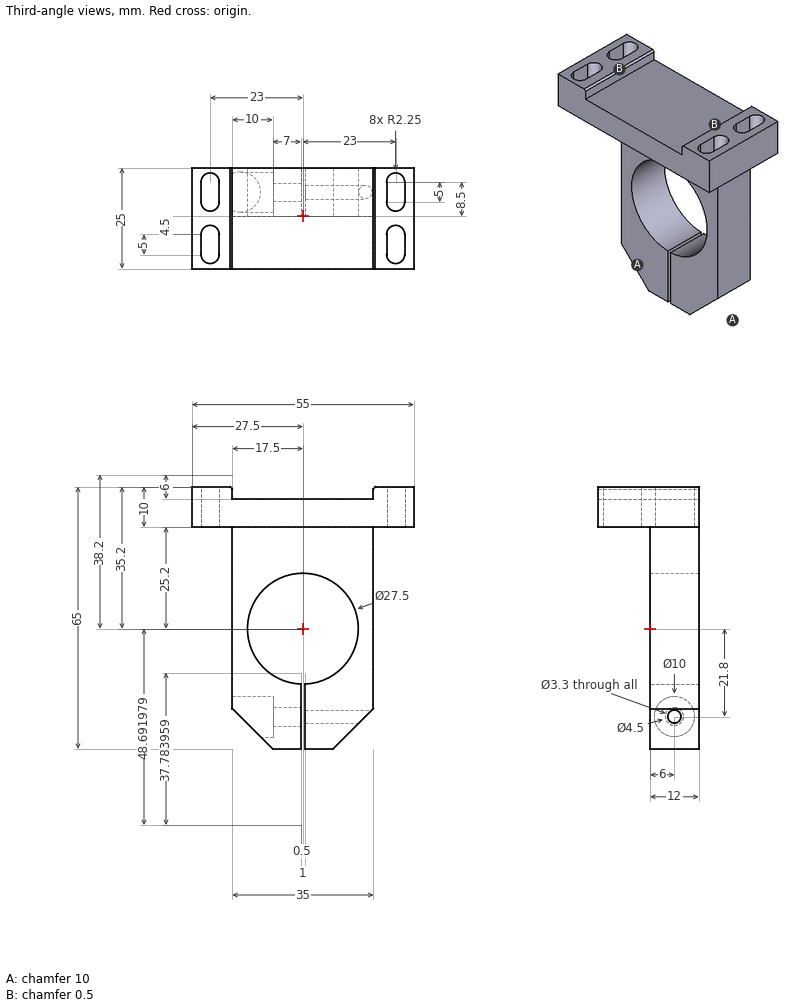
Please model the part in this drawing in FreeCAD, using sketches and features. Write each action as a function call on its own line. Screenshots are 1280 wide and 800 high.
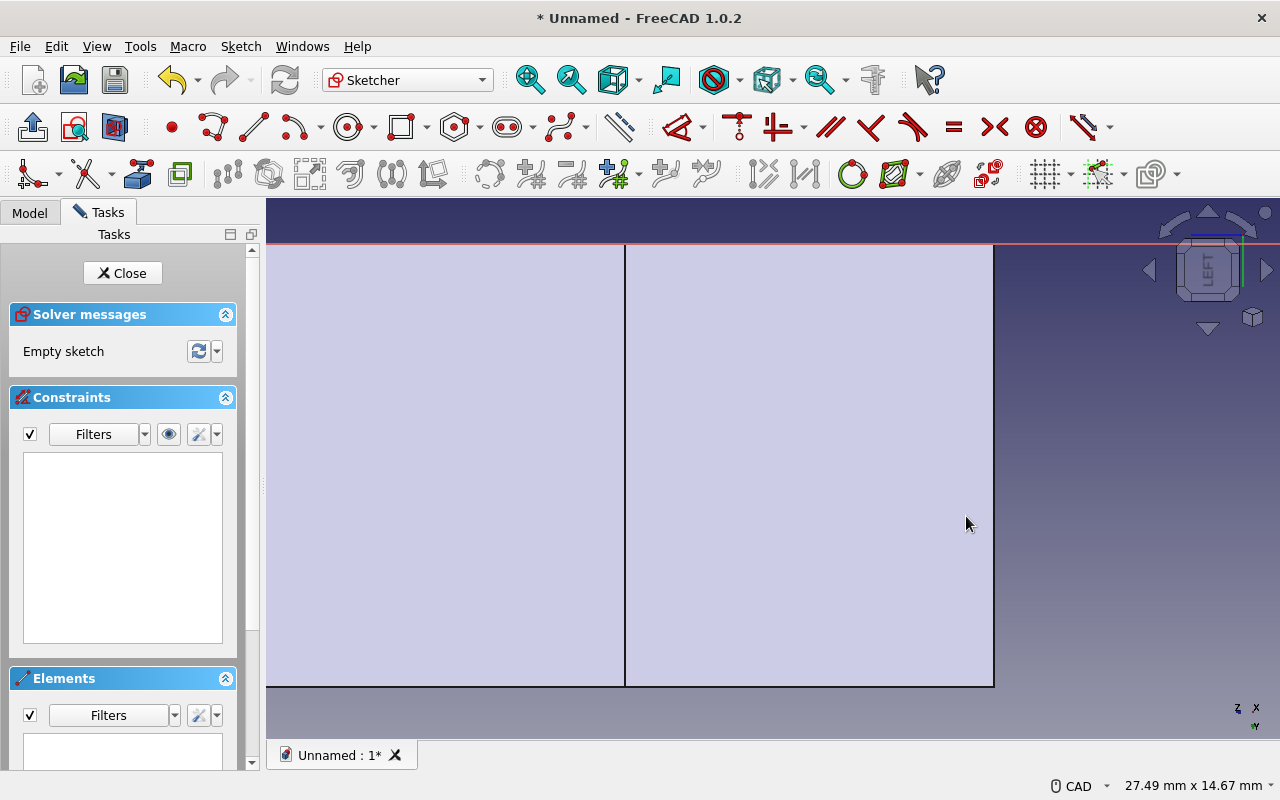
key(g)
key(c)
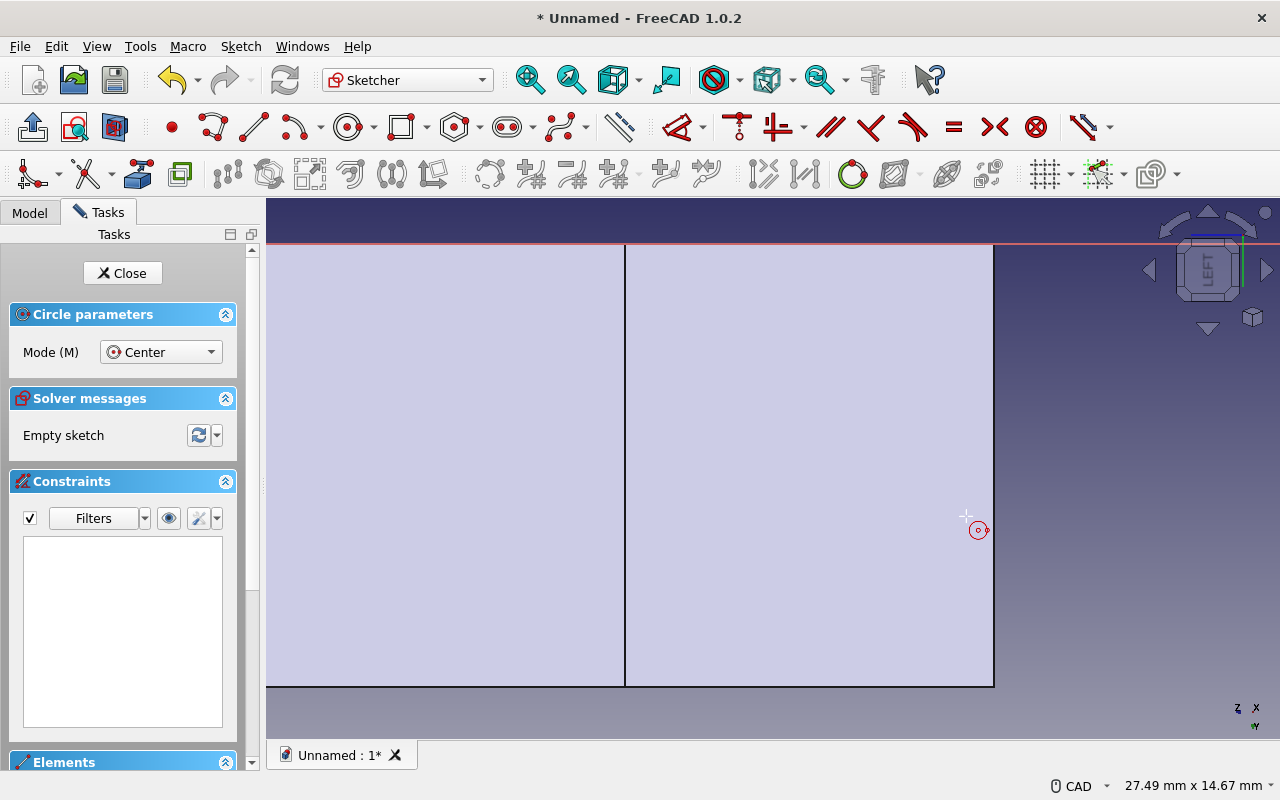
click(699, 465)
click(829, 335)
key(Escape)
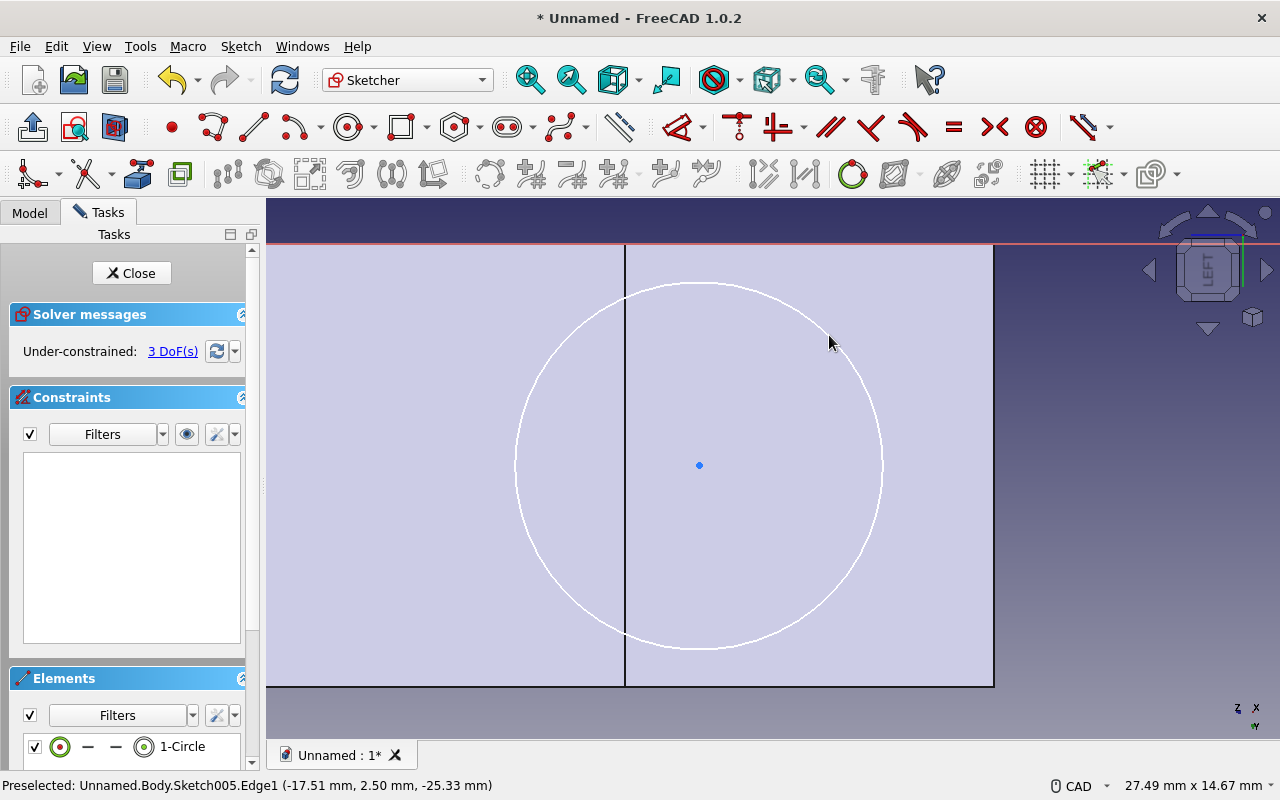
key(d)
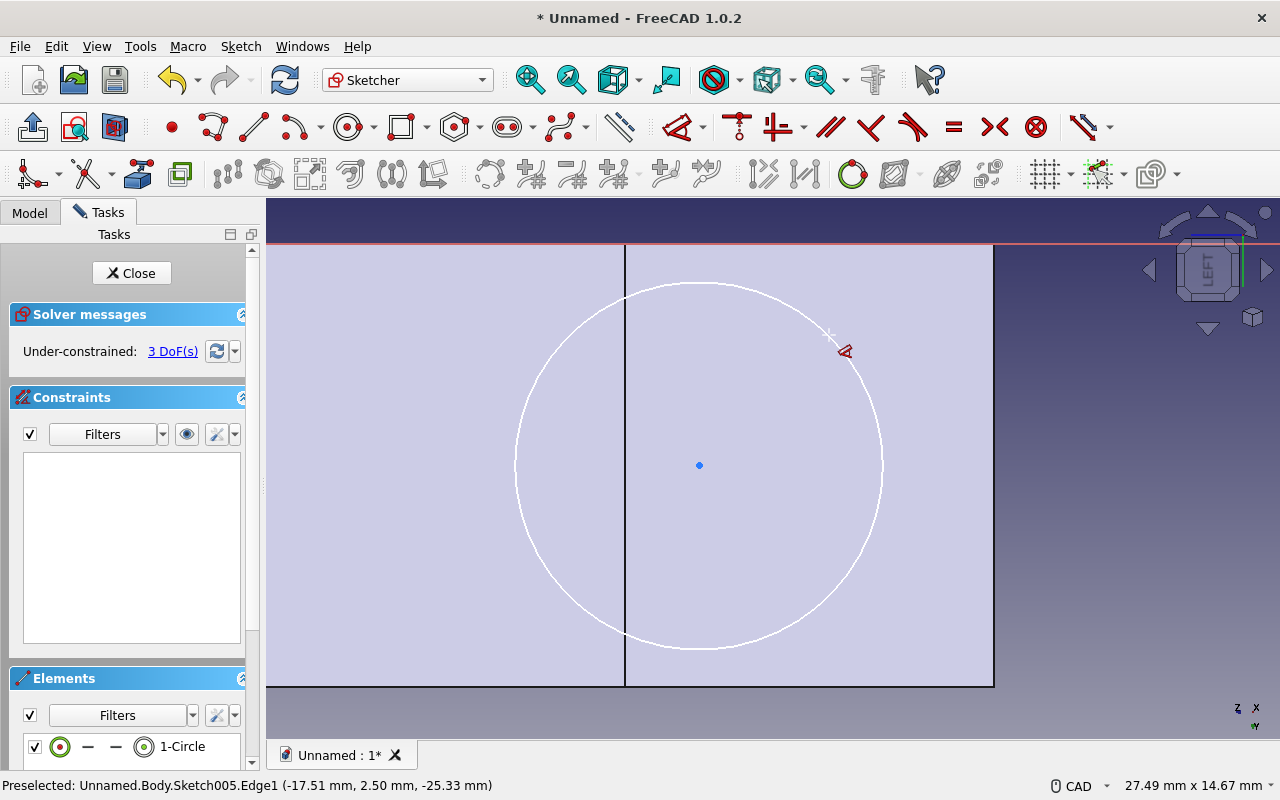
click(829, 336)
click(852, 313)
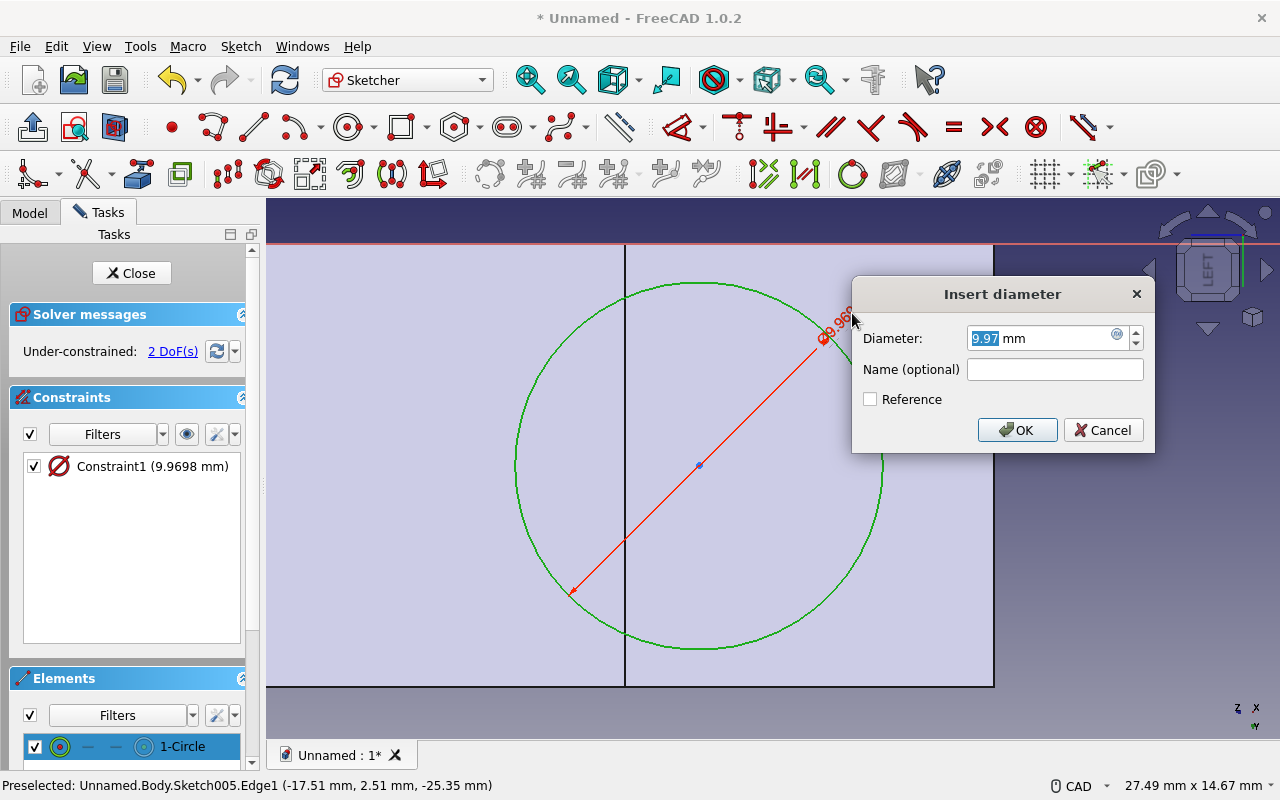
text(10)
key(Return)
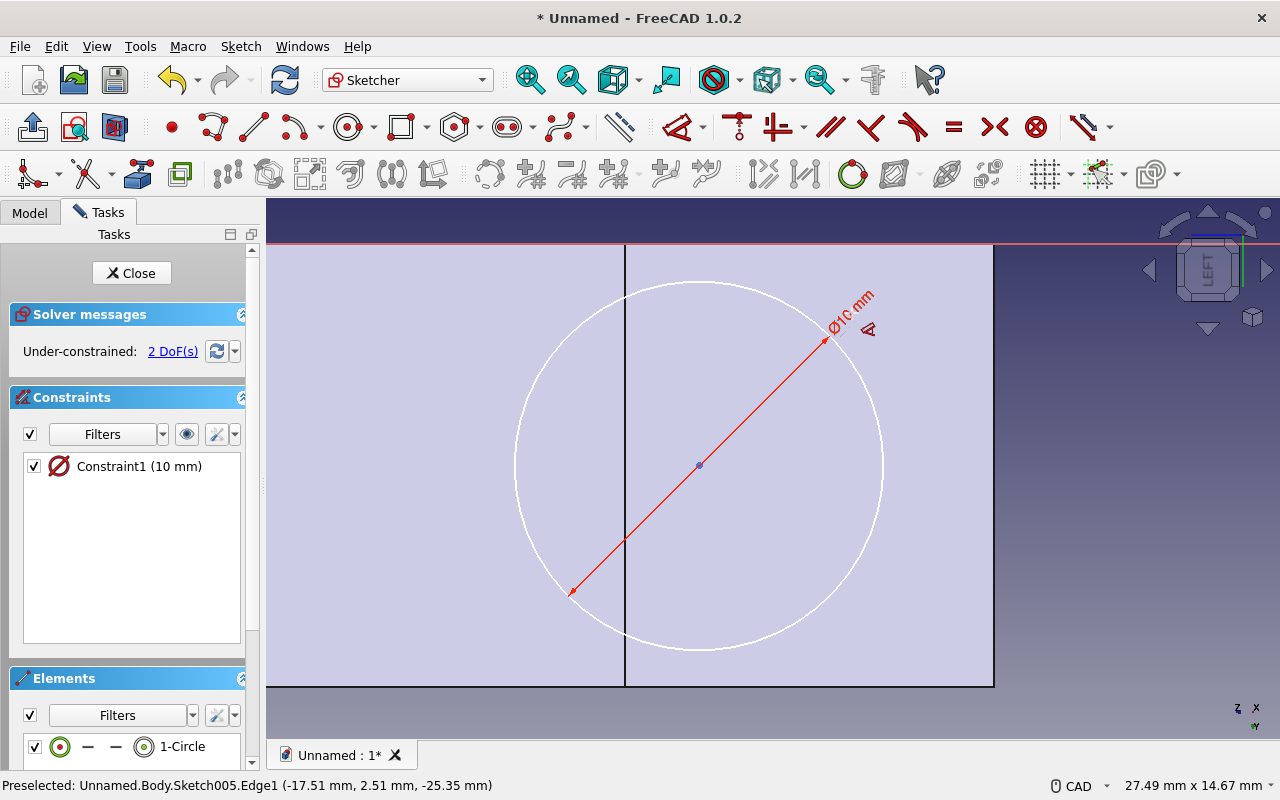
click(699, 466)
click(733, 355)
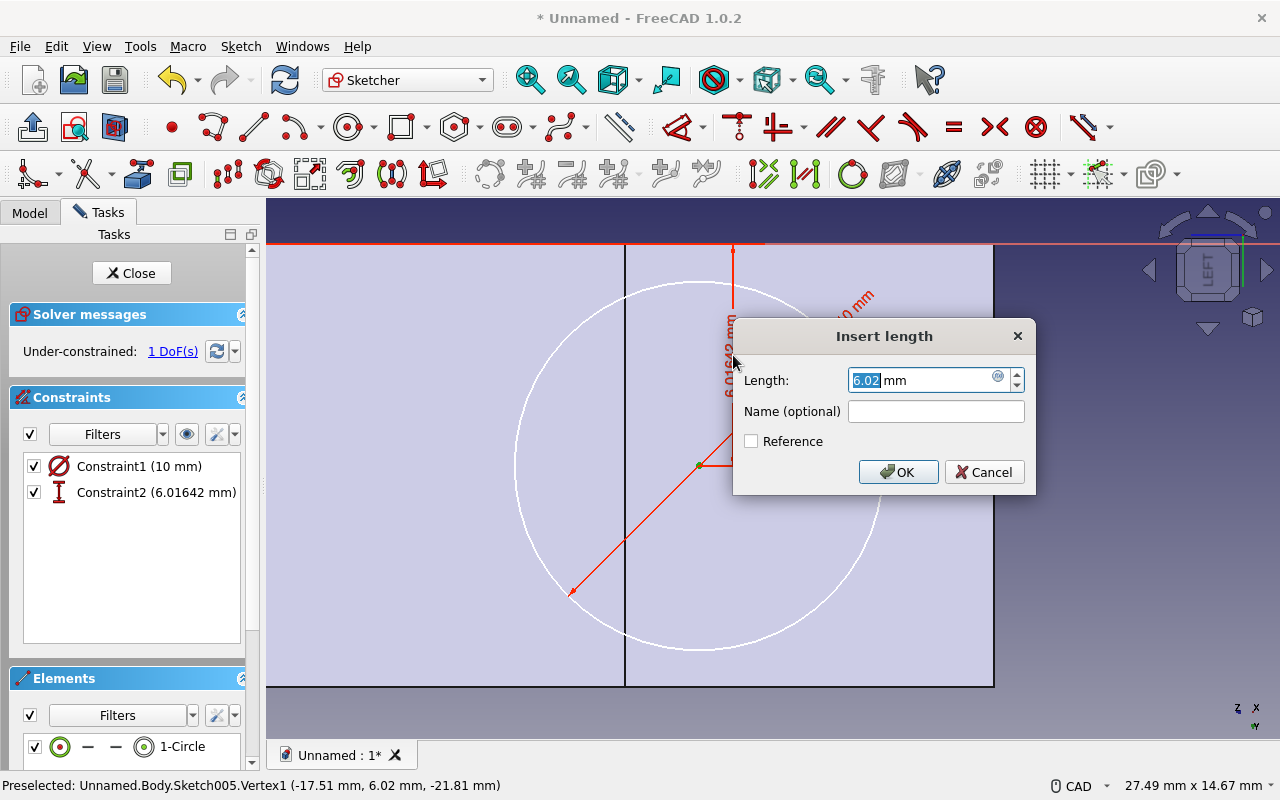
text(6)
key(Return)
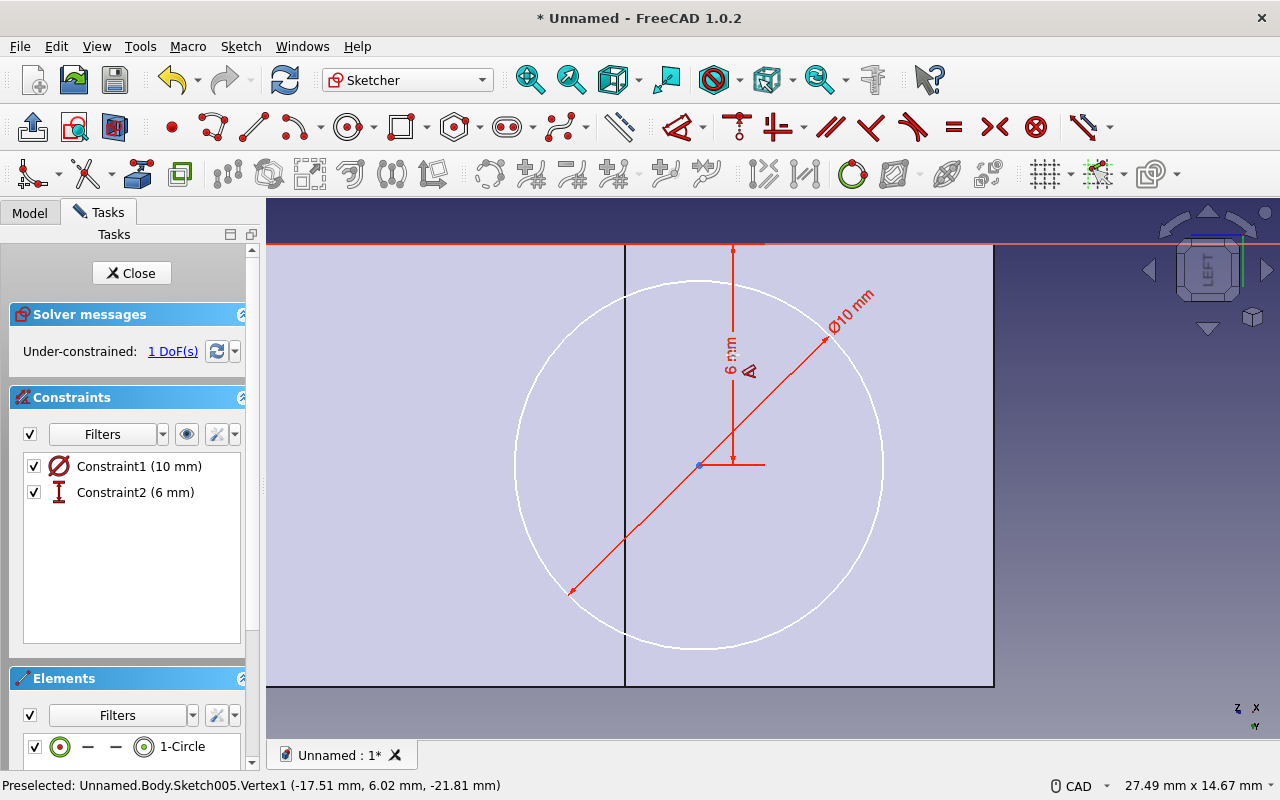
click(699, 465)
click(497, 499)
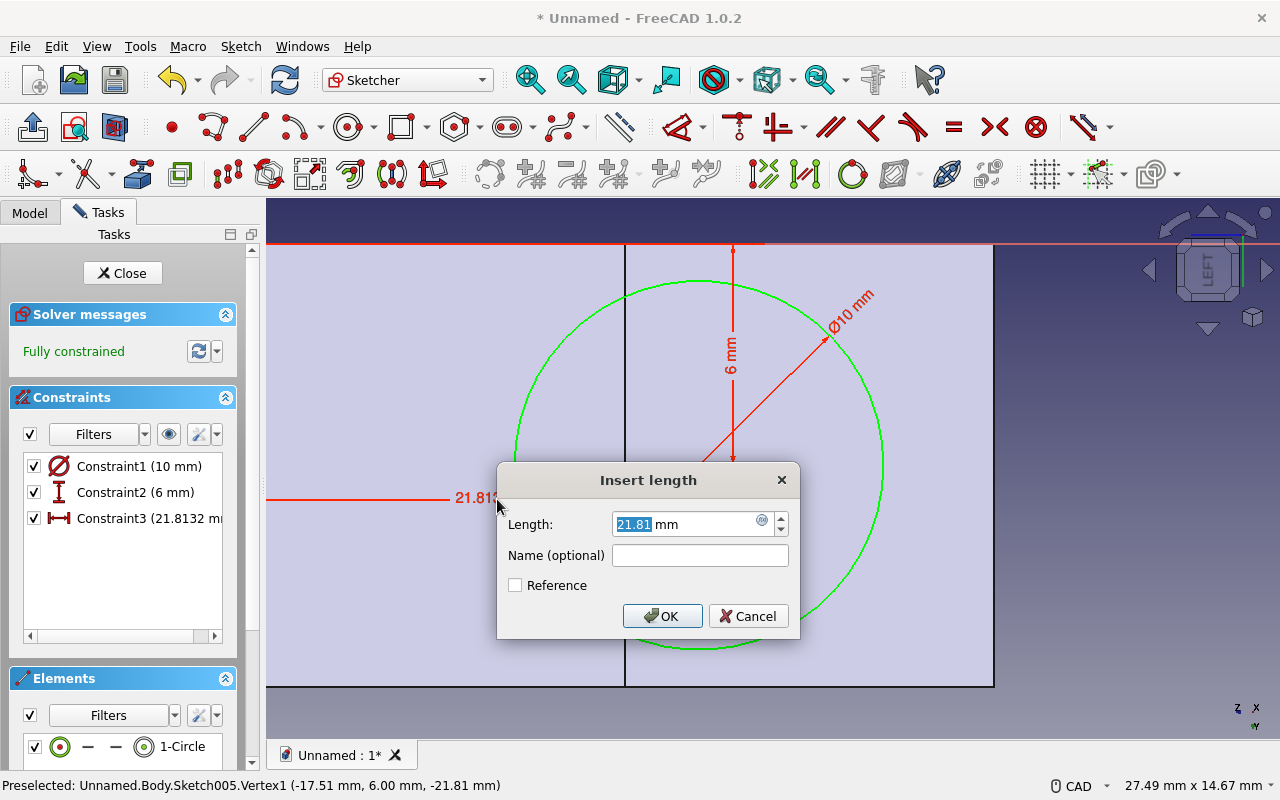
text(21.8)
key(Return)
key(Escape)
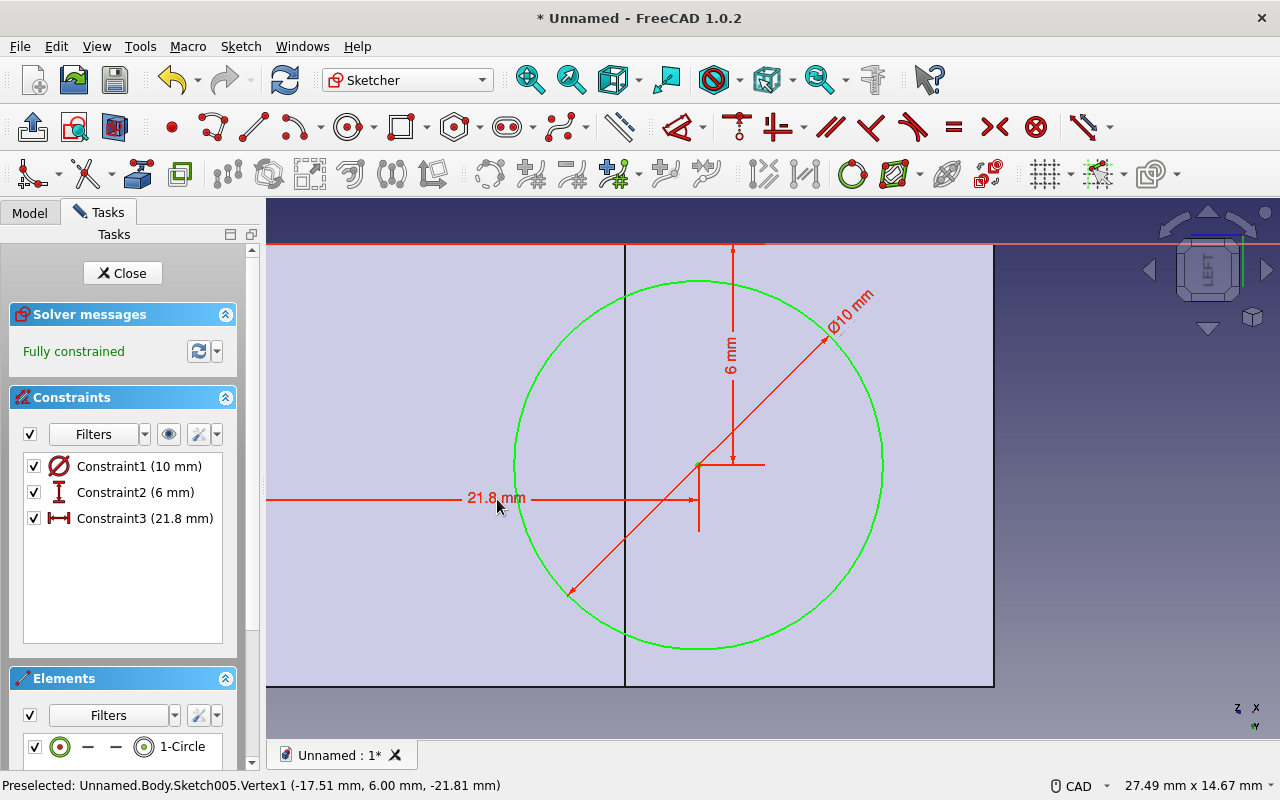
click(123, 273)